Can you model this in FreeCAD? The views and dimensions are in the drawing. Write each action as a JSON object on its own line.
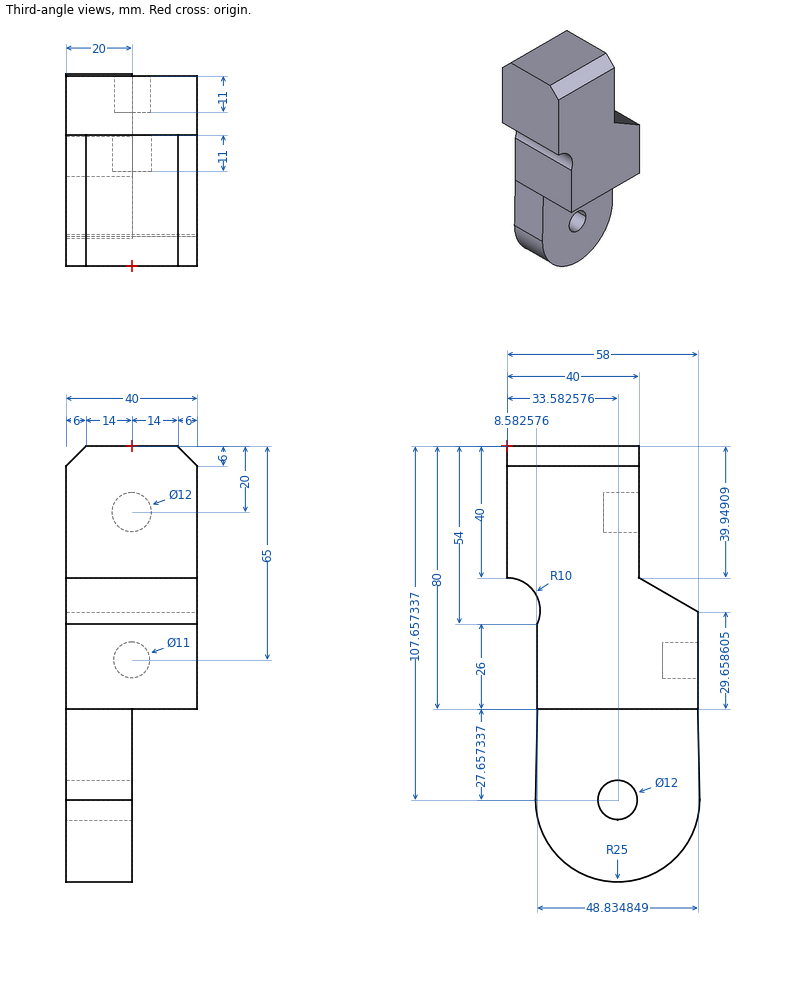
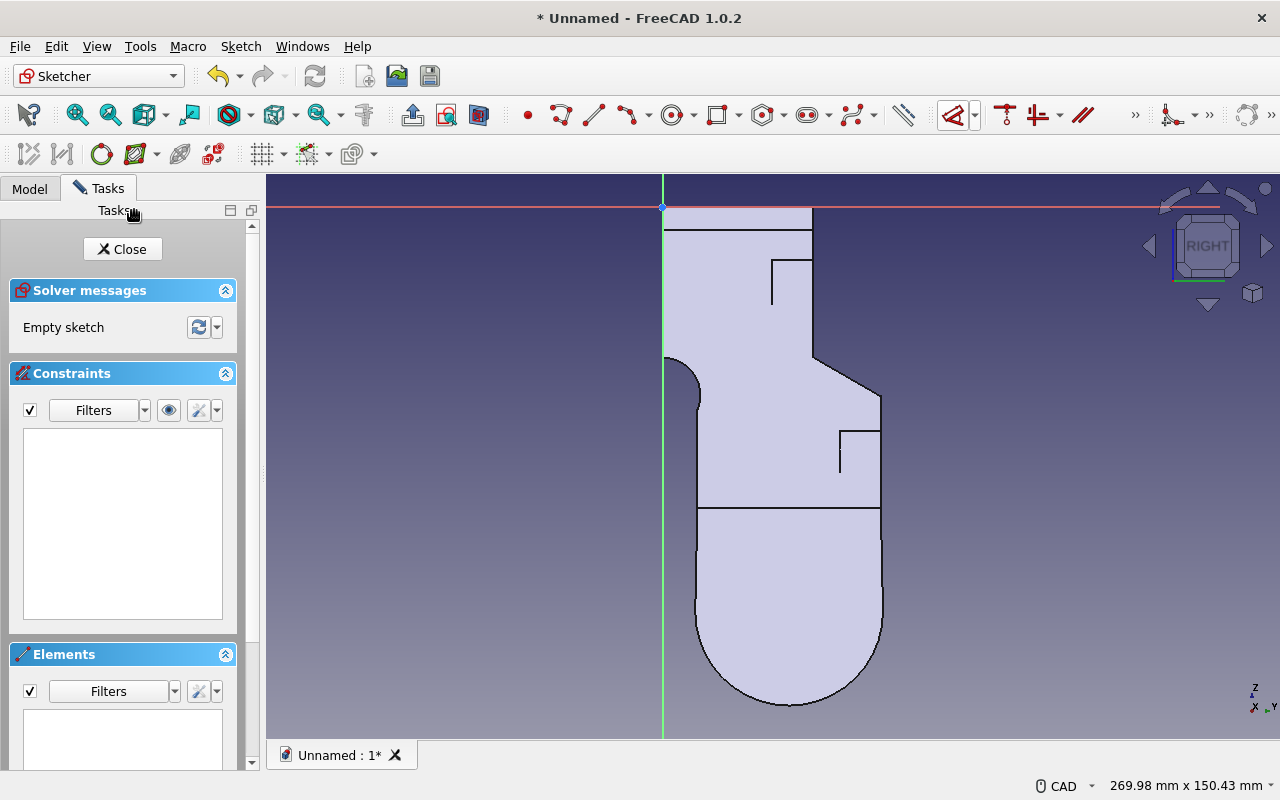
{"action": "scroll", "coordinate": [802, 636], "scroll_direction": "up", "scroll_amount": 10}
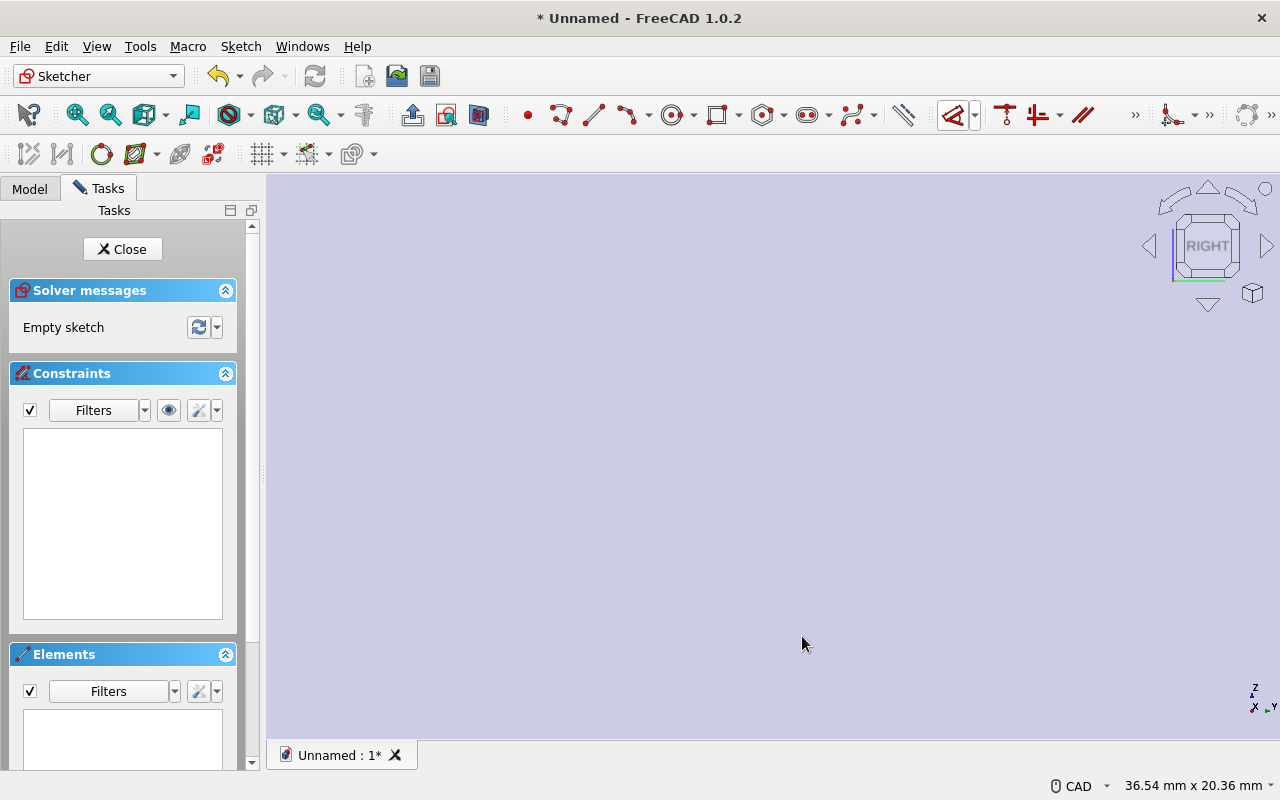
{"action": "key", "text": "g c"}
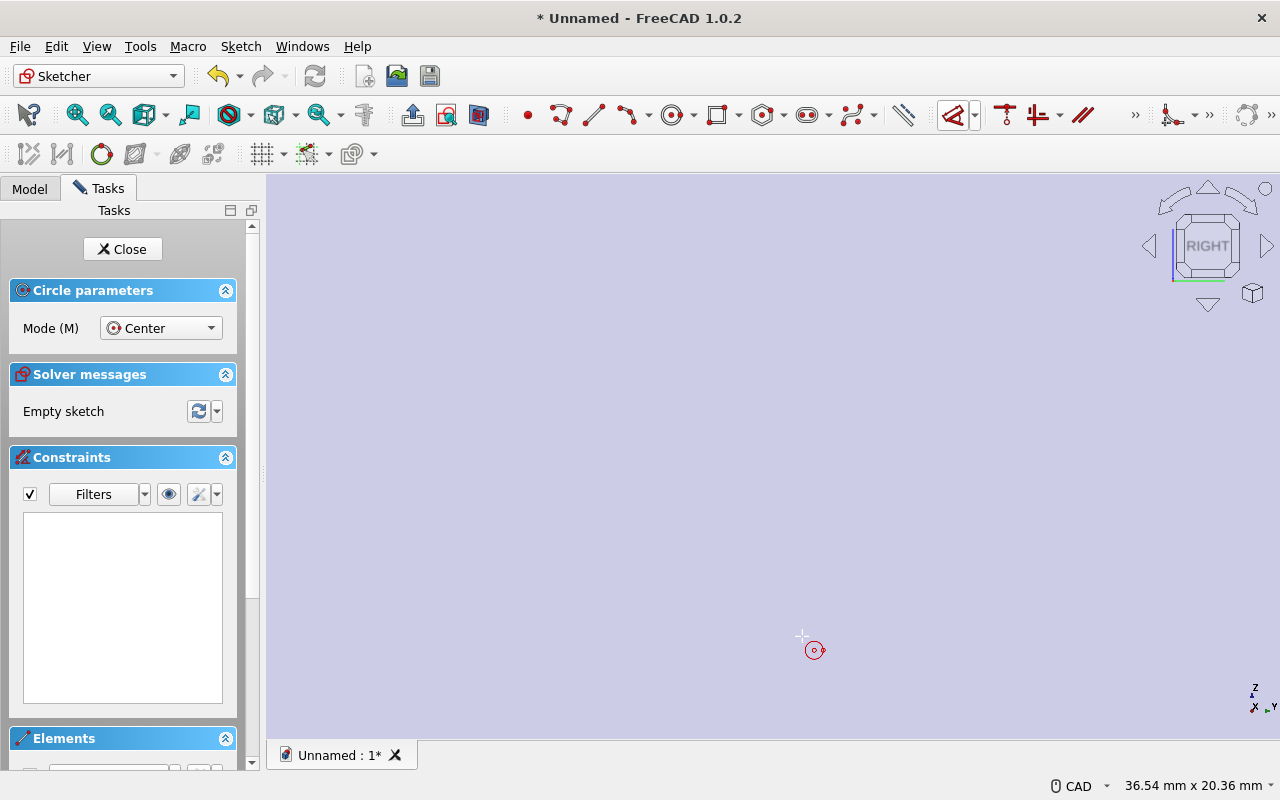
{"action": "left_click", "coordinate": [703, 451]}
{"action": "mouse_move", "coordinate": [821, 334]}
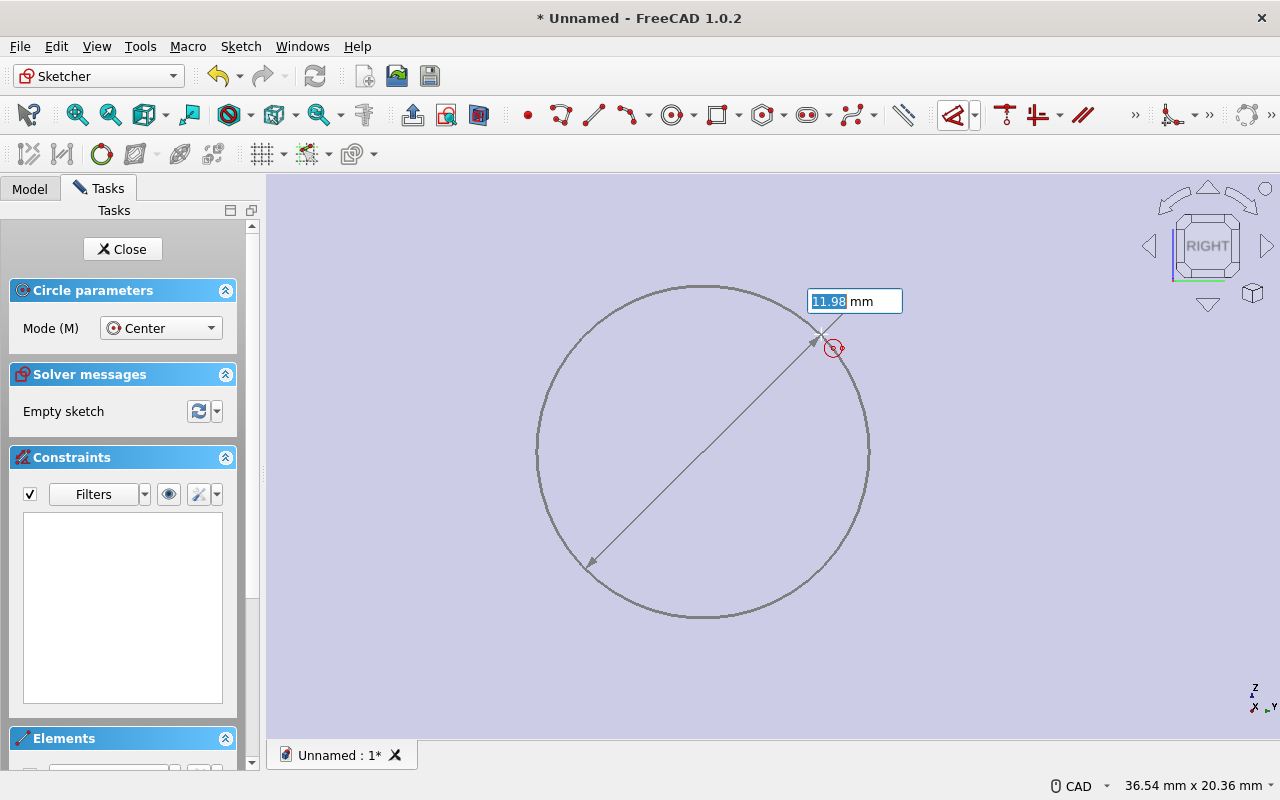
{"action": "type", "text": "12"}
{"action": "key", "text": "Return"}
{"action": "key", "text": "Escape"}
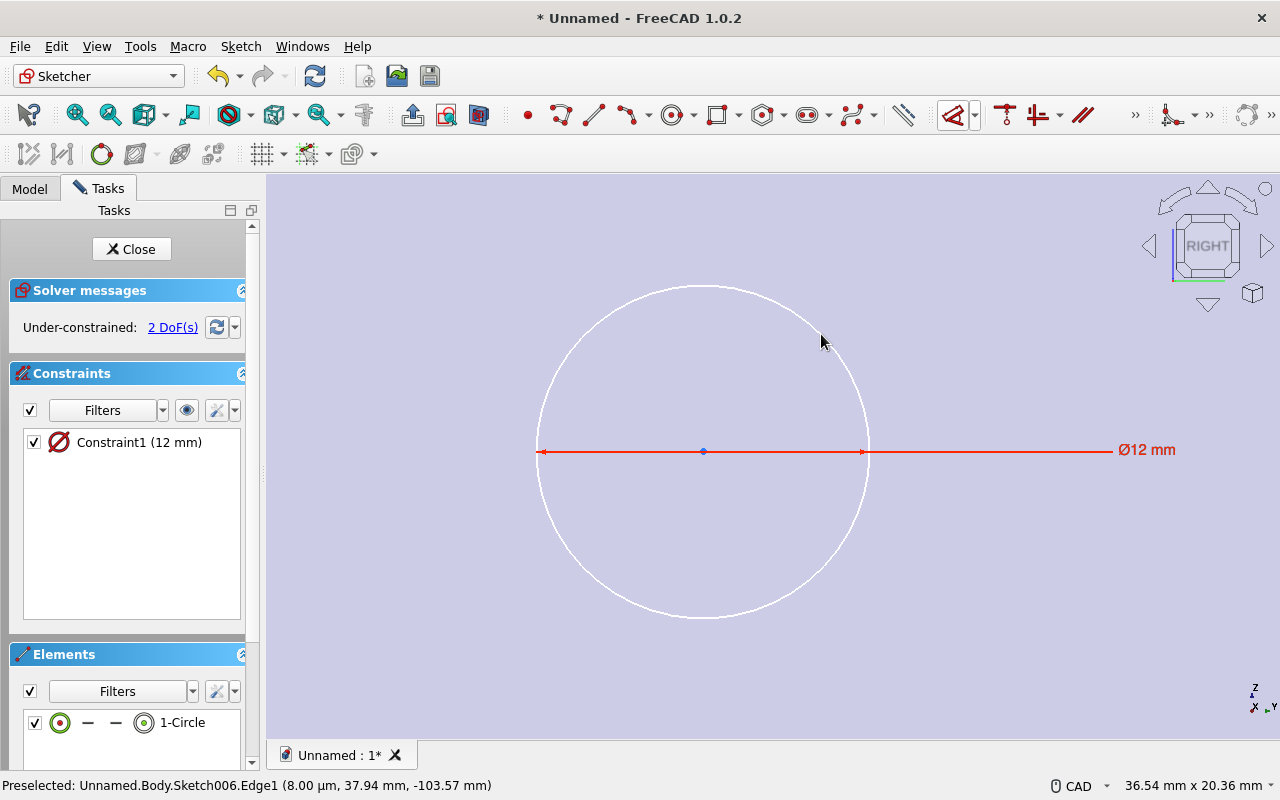
{"action": "left_click", "coordinate": [703, 452]}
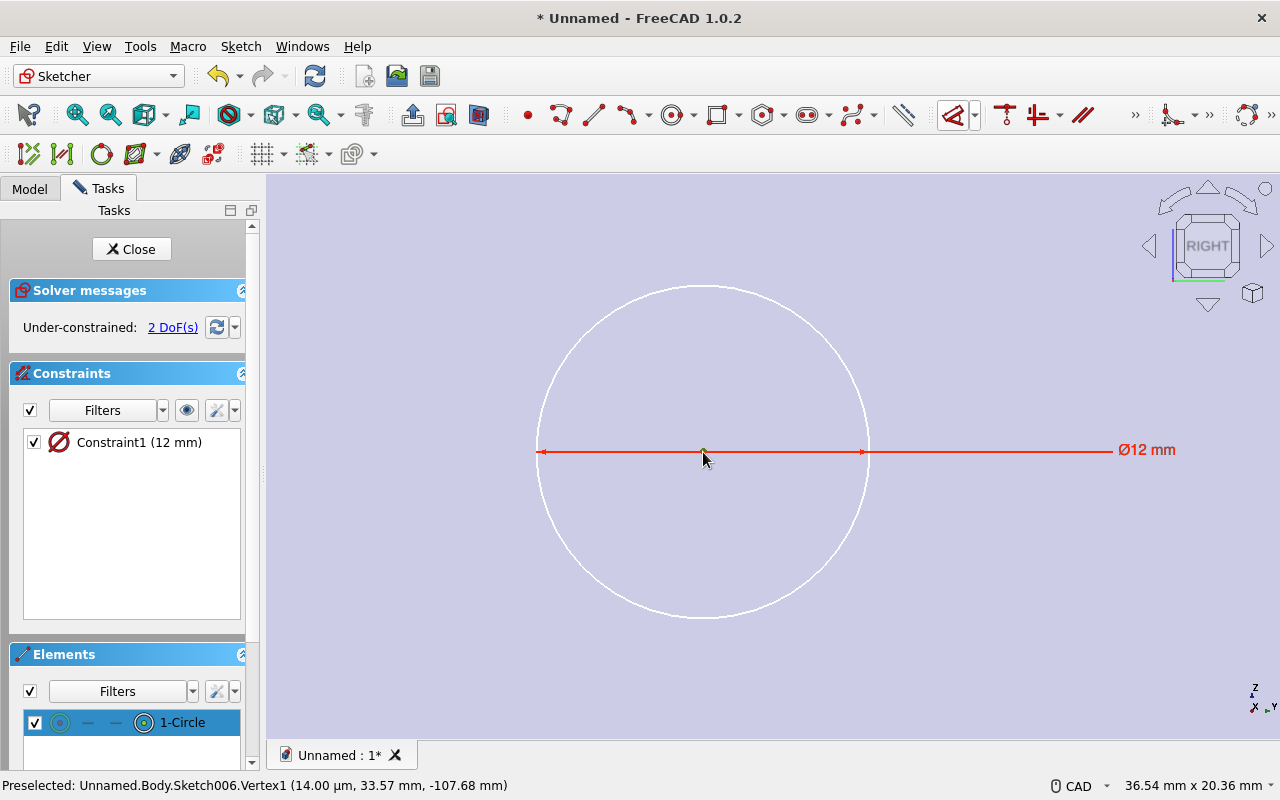
{"action": "key", "text": "l"}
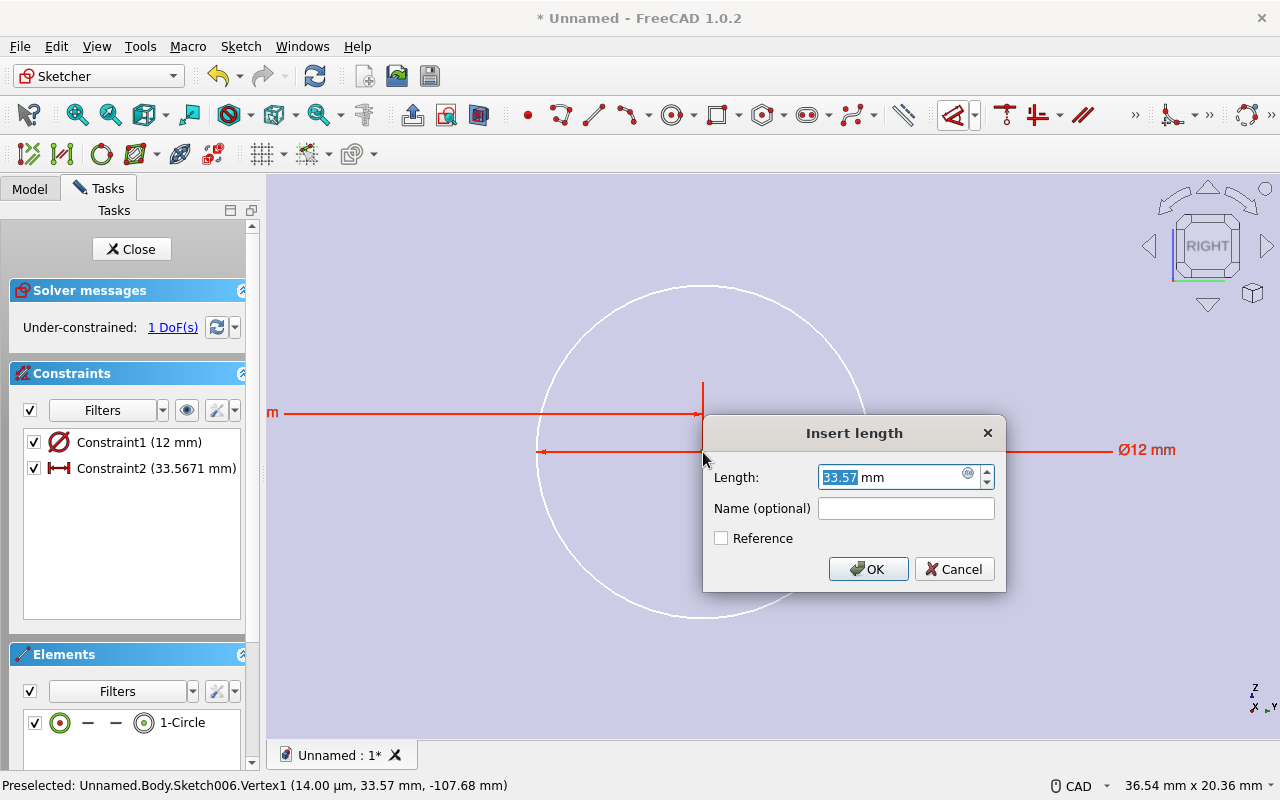
{"action": "type", "text": "33.582576"}
{"action": "key", "text": "Return"}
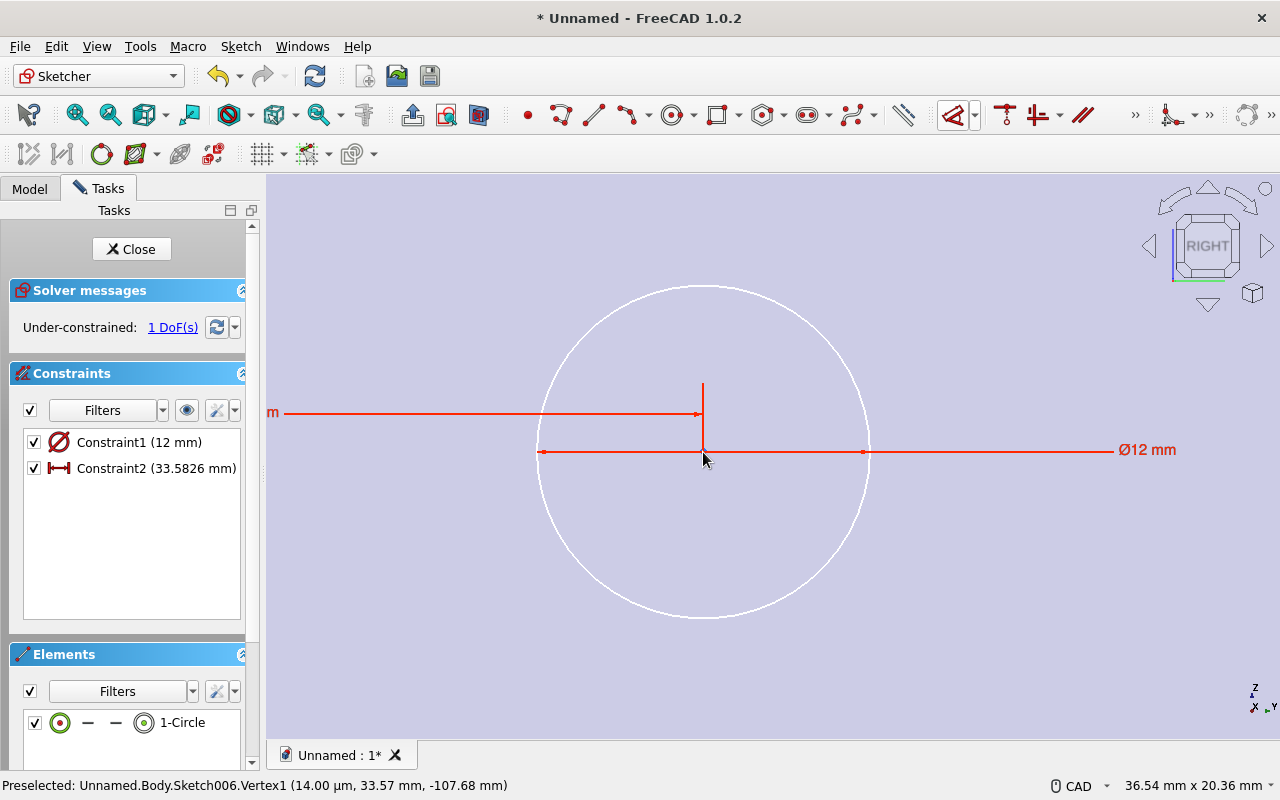
{"action": "left_click", "coordinate": [703, 452]}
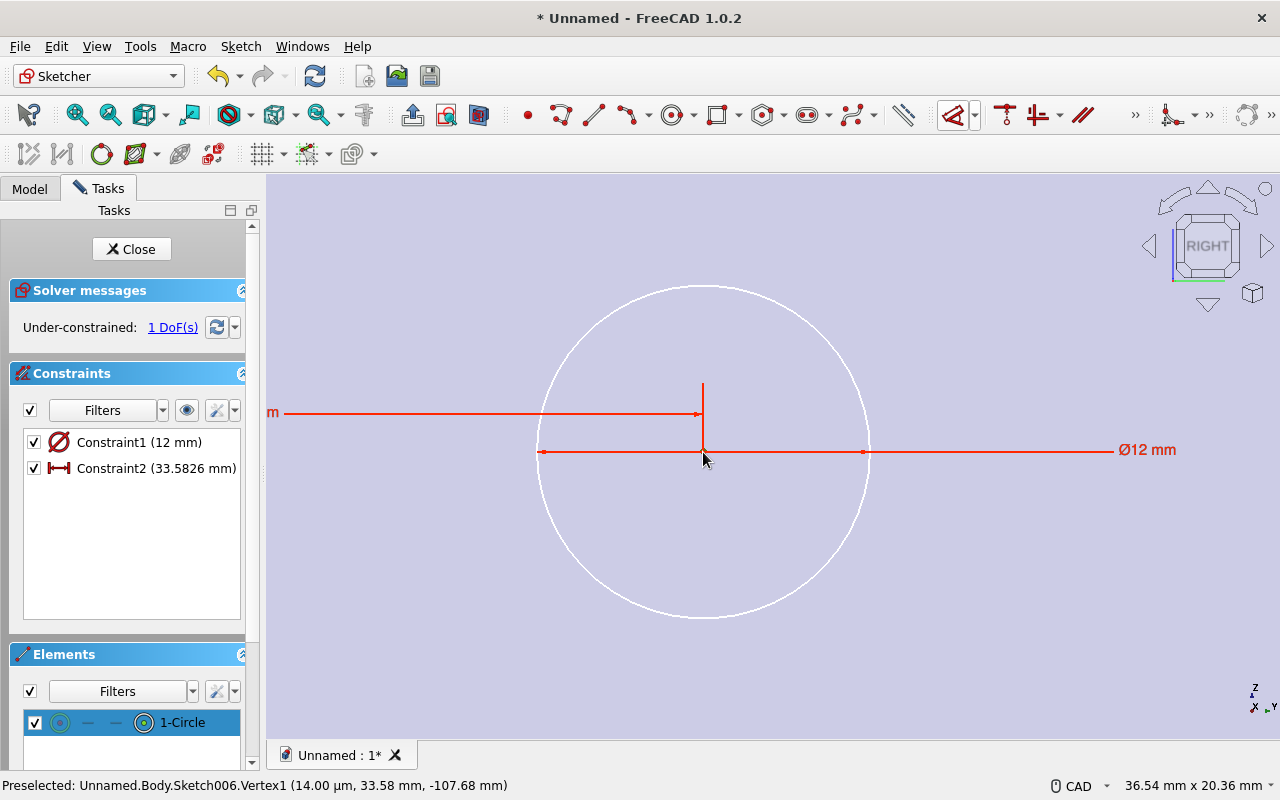
{"action": "key", "text": "i"}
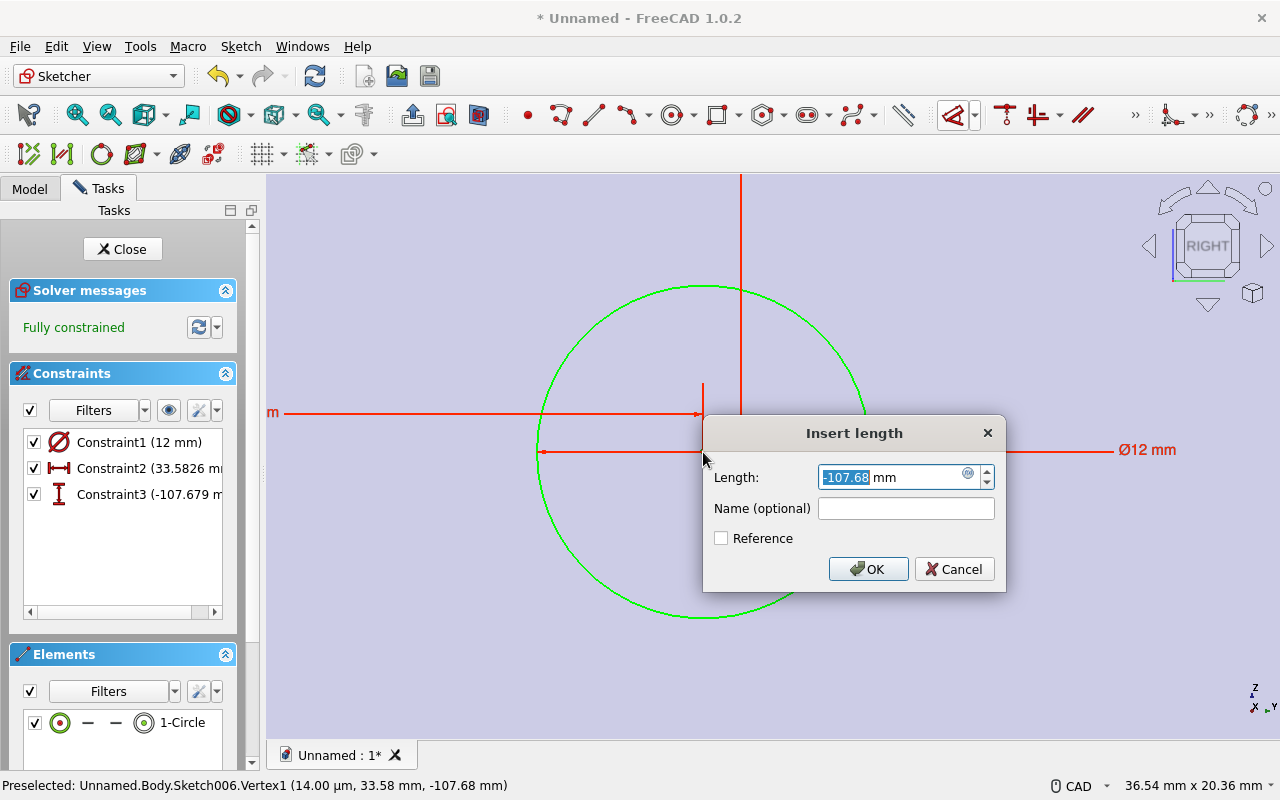
{"action": "type", "text": "-107.657337"}
{"action": "key", "text": "Return"}